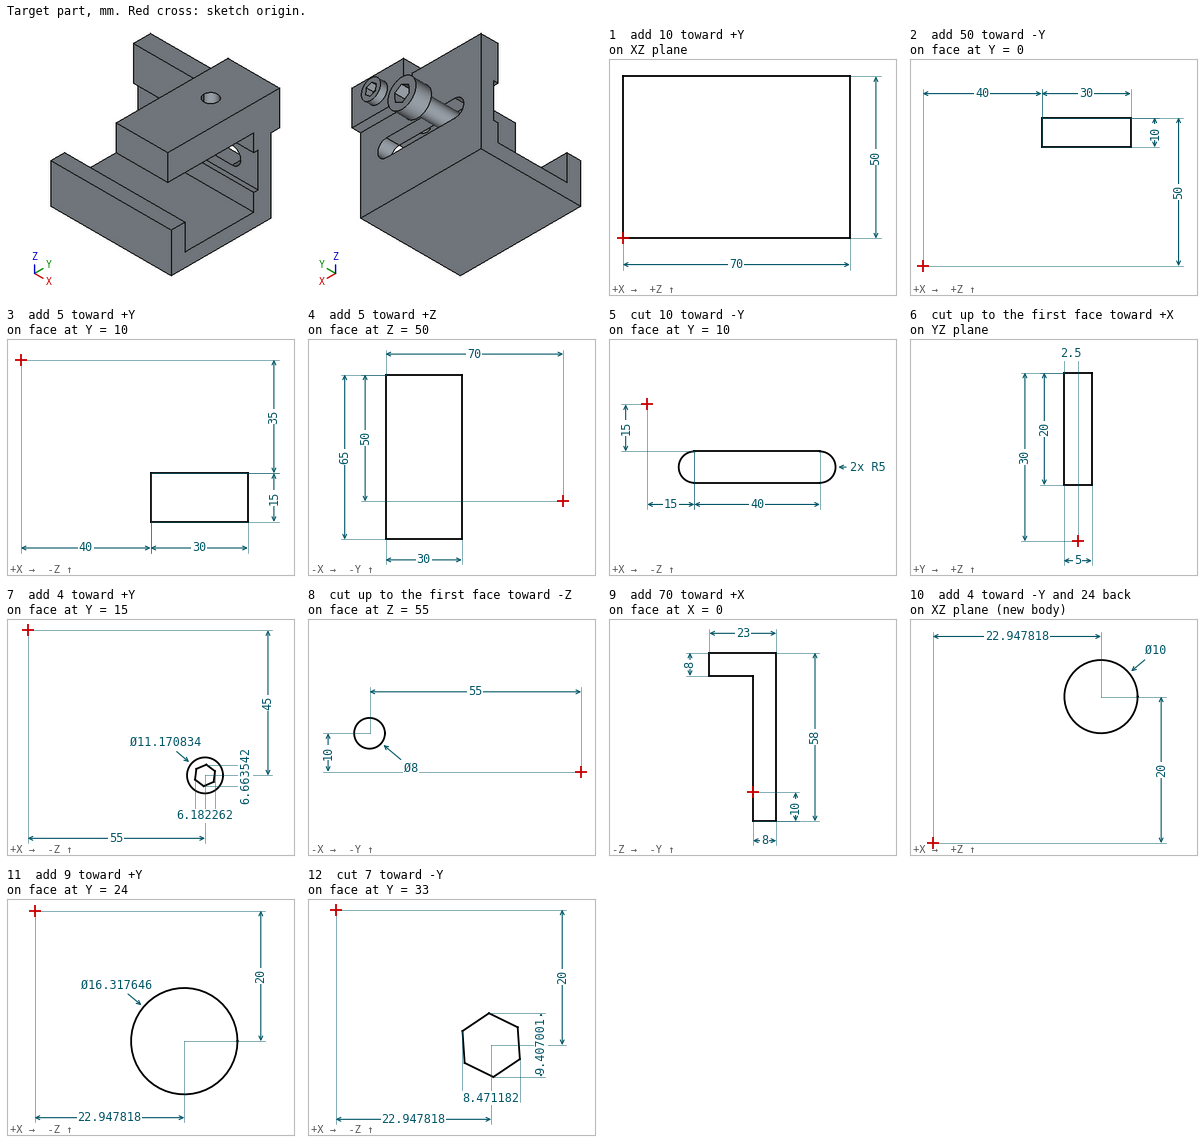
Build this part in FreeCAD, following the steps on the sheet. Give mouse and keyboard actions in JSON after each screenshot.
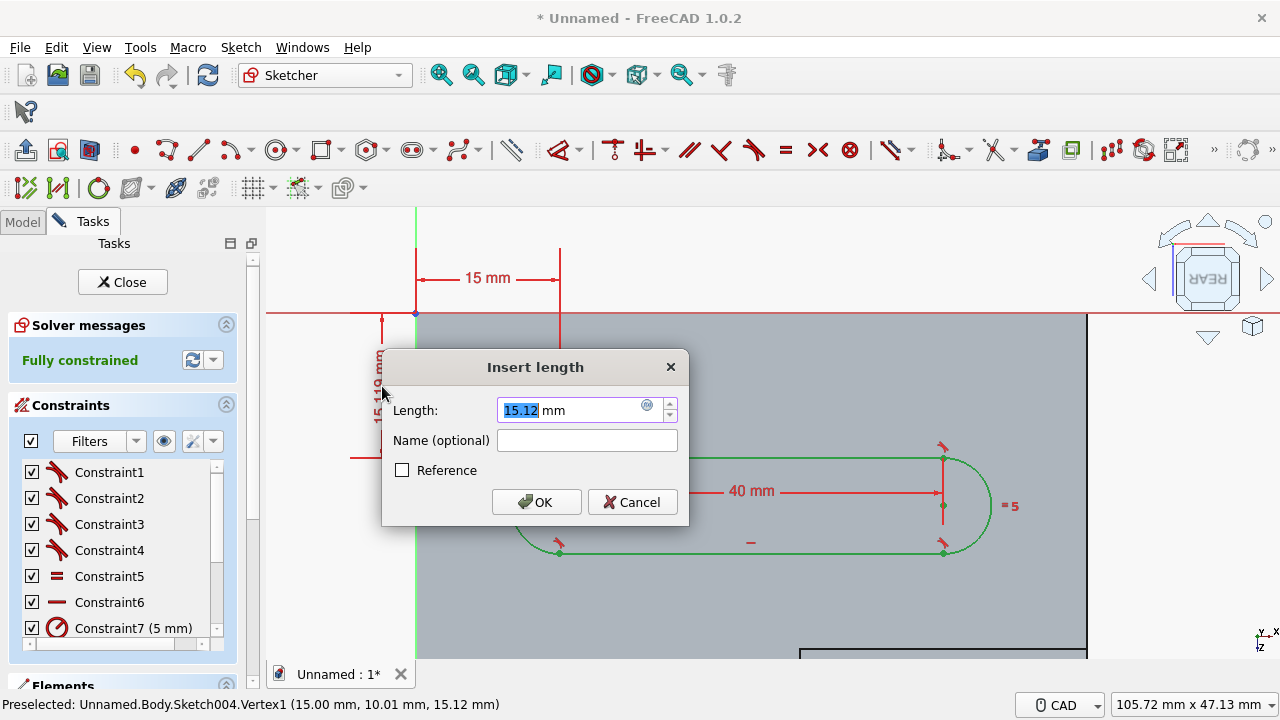
{"action": "type", "text": "15"}
{"action": "key", "text": "Return"}
{"action": "key", "text": "Escape"}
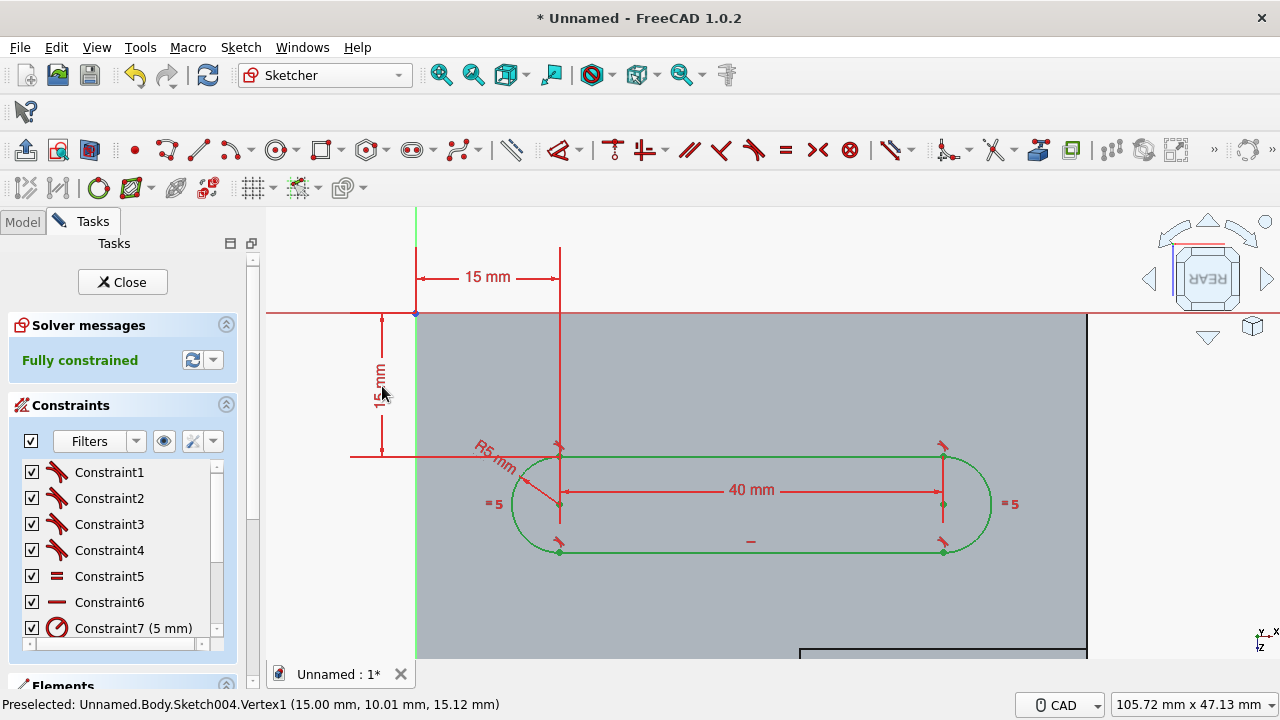
{"action": "left_click", "coordinate": [123, 282]}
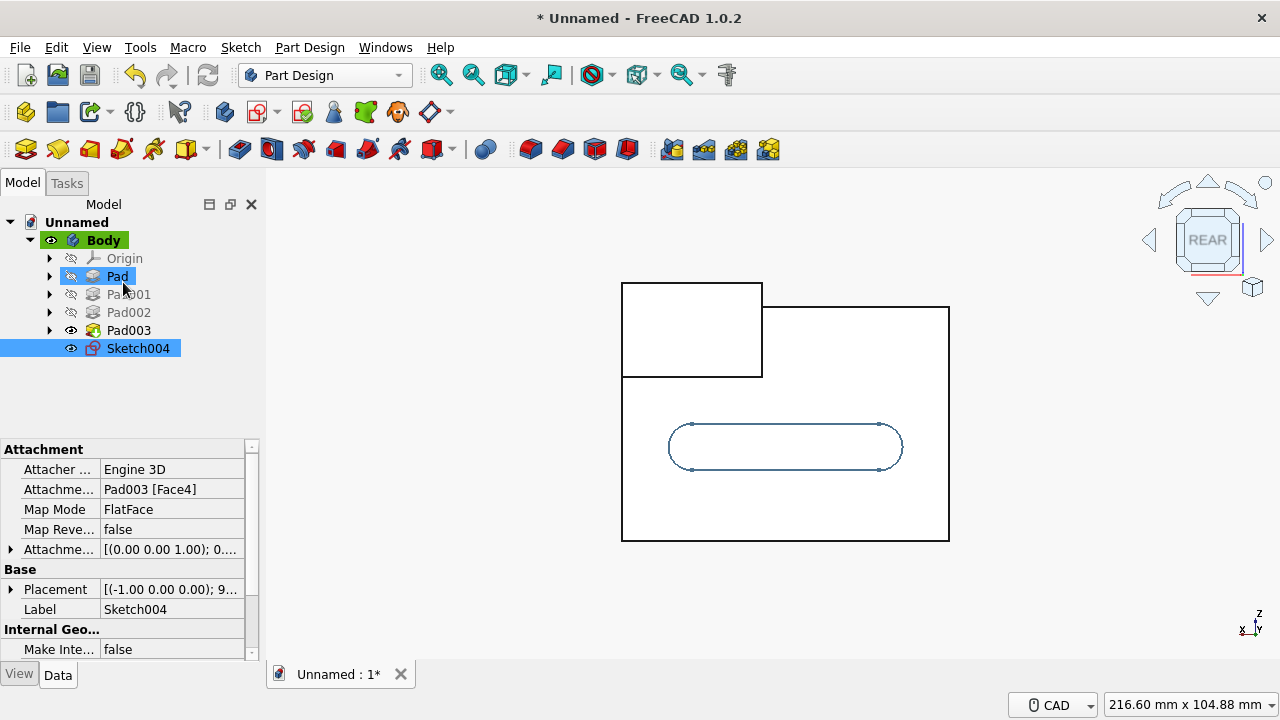
{"action": "left_click", "coordinate": [240, 150]}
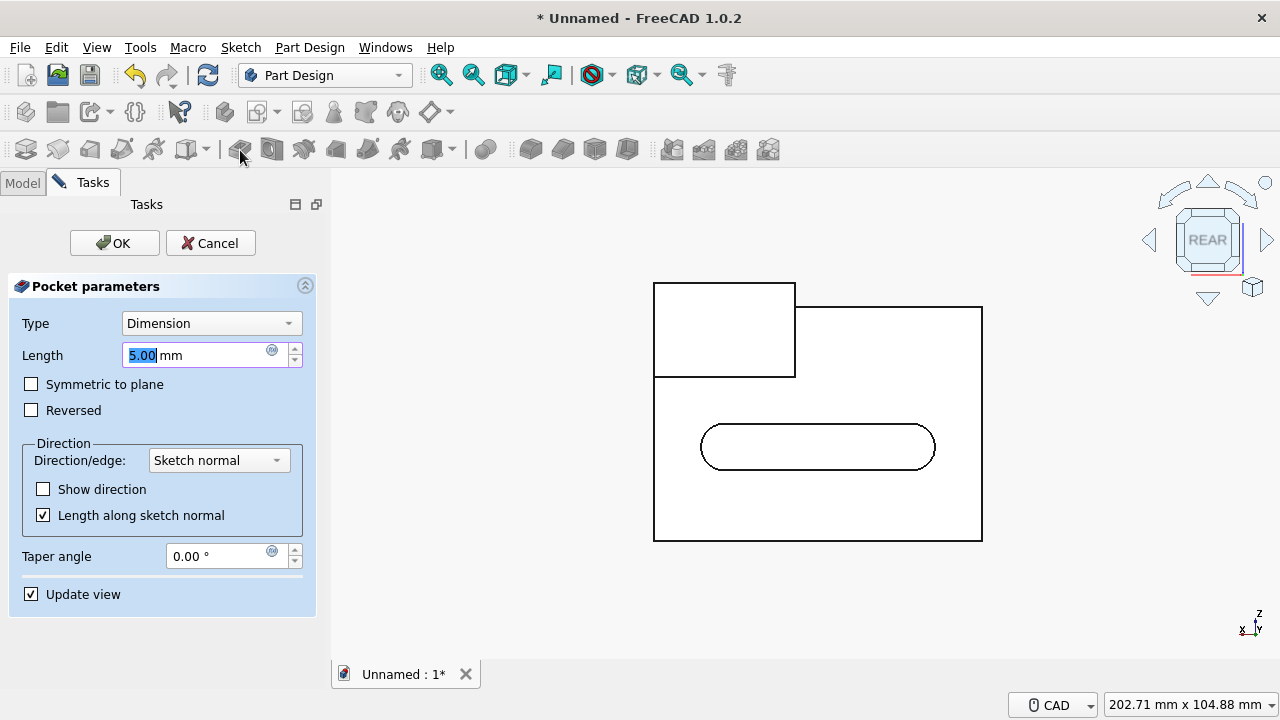
{"action": "type", "text": "10"}
{"action": "key", "text": "Tab"}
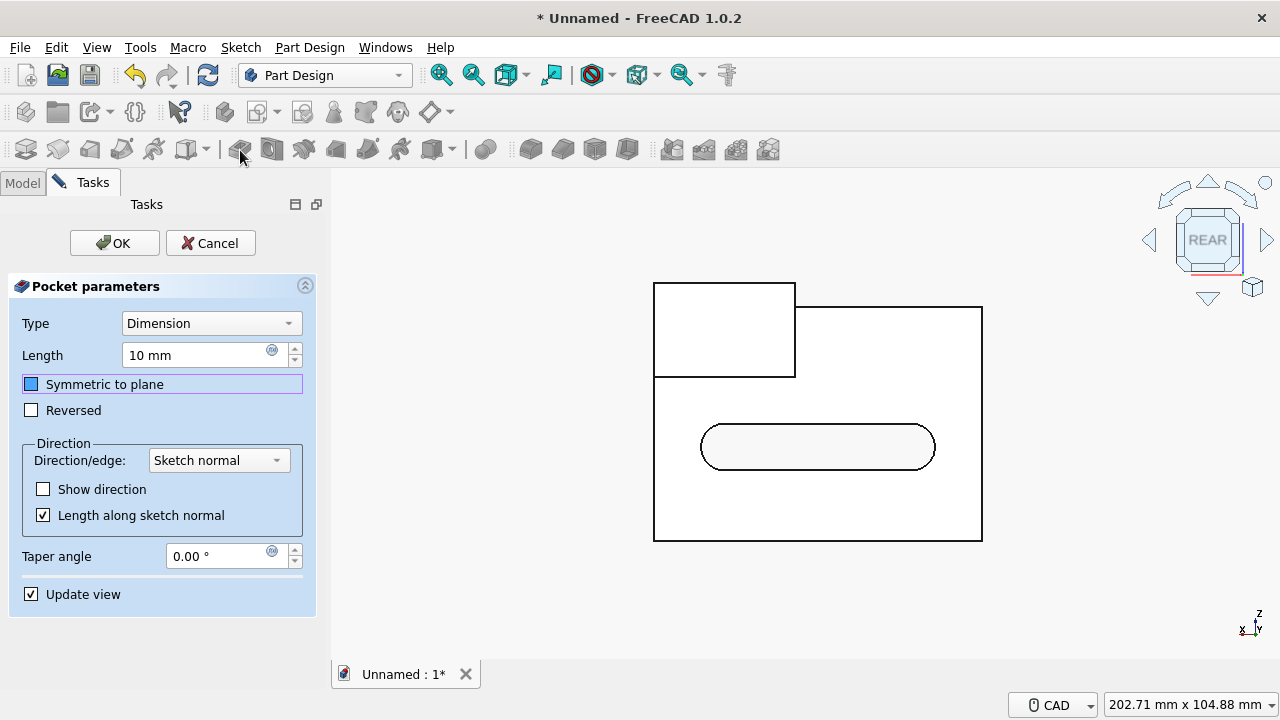
{"action": "left_click", "coordinate": [115, 243]}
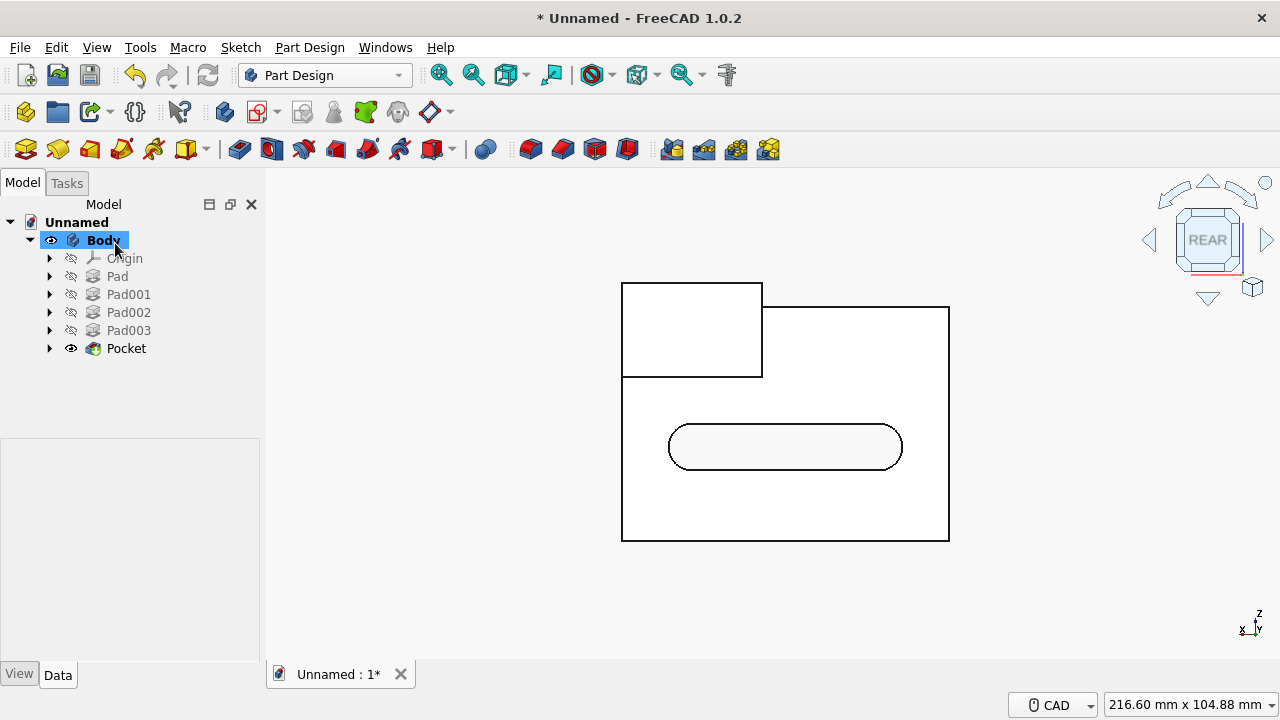
{"action": "left_click", "coordinate": [258, 112]}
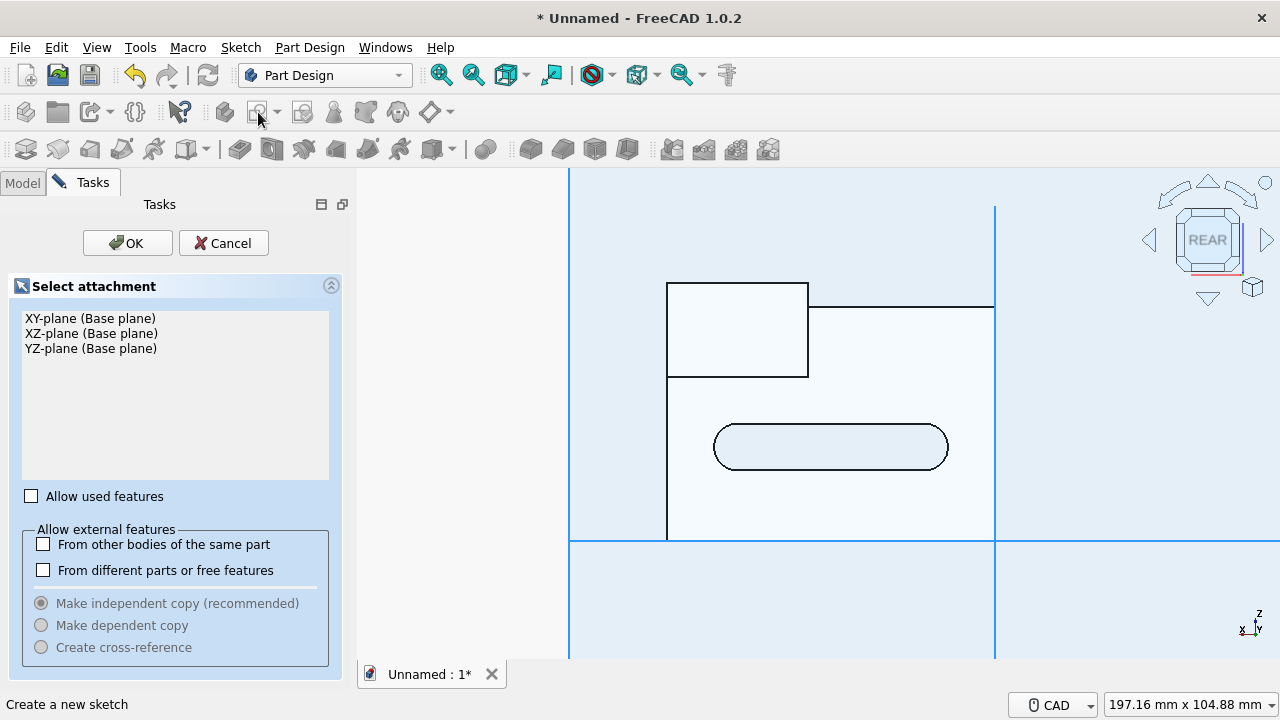
{"action": "left_click", "coordinate": [82, 348]}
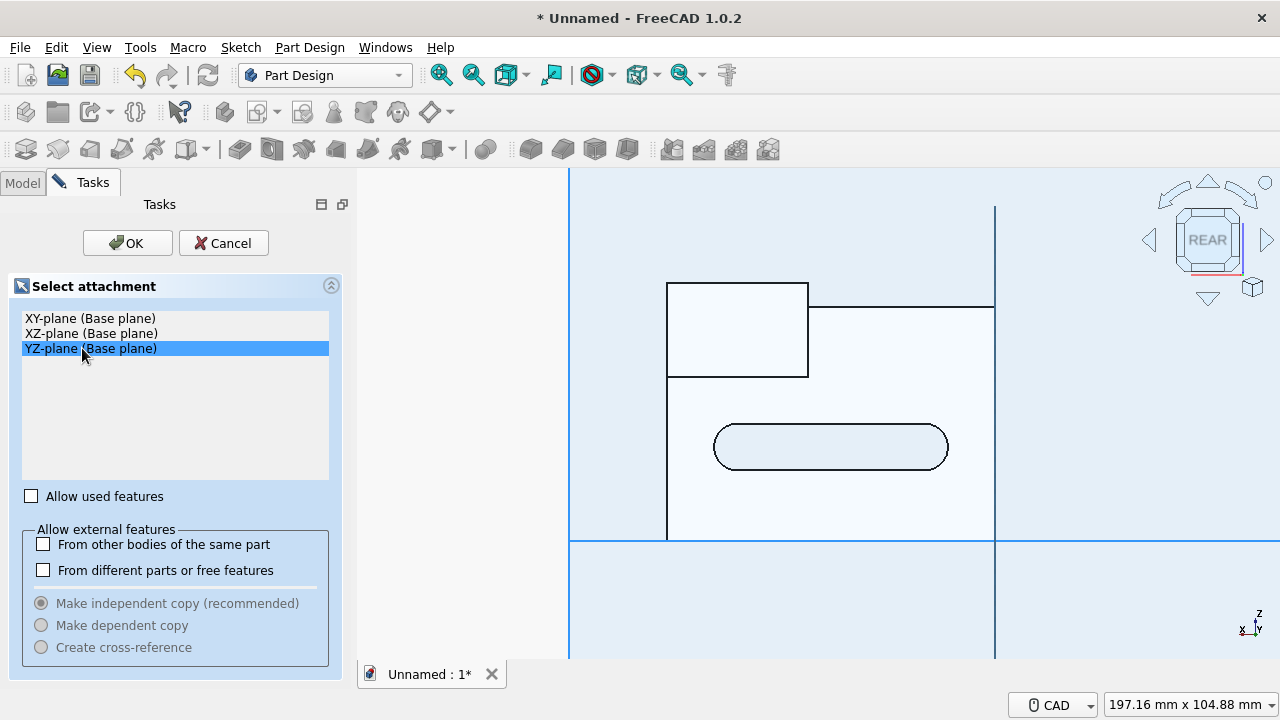
{"action": "left_click", "coordinate": [128, 243]}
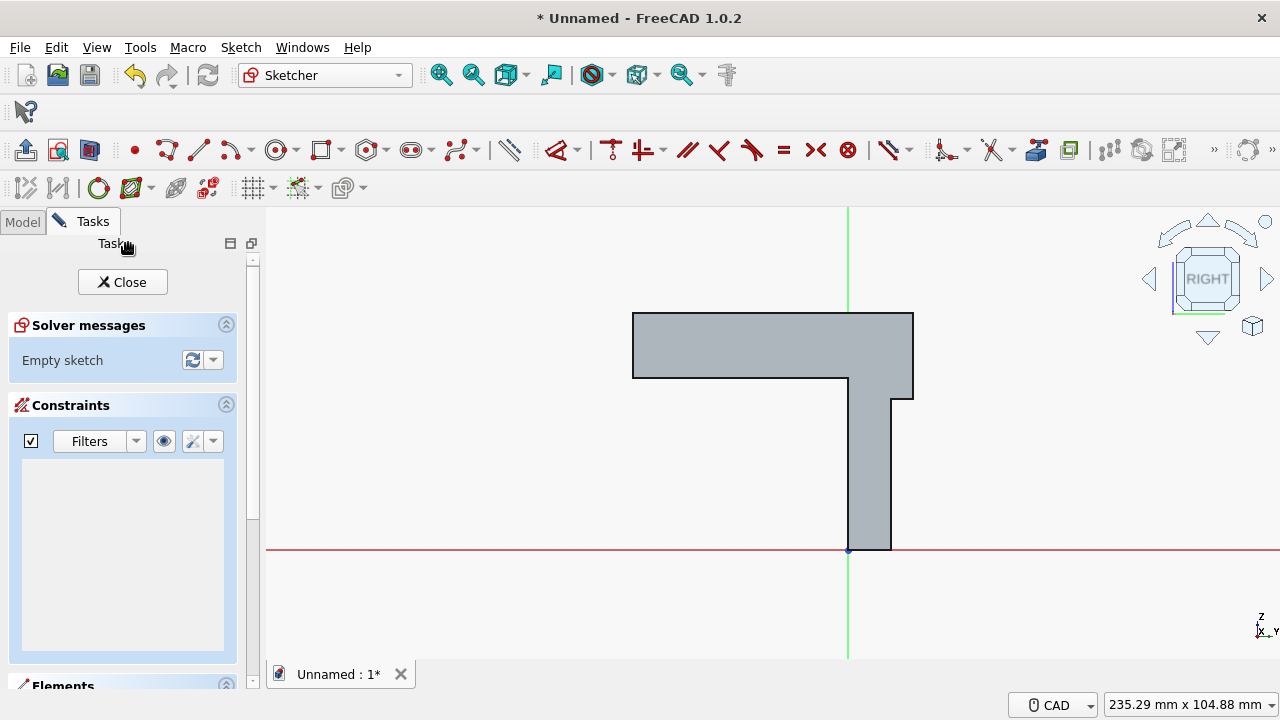
{"action": "left_click", "coordinate": [90, 150]}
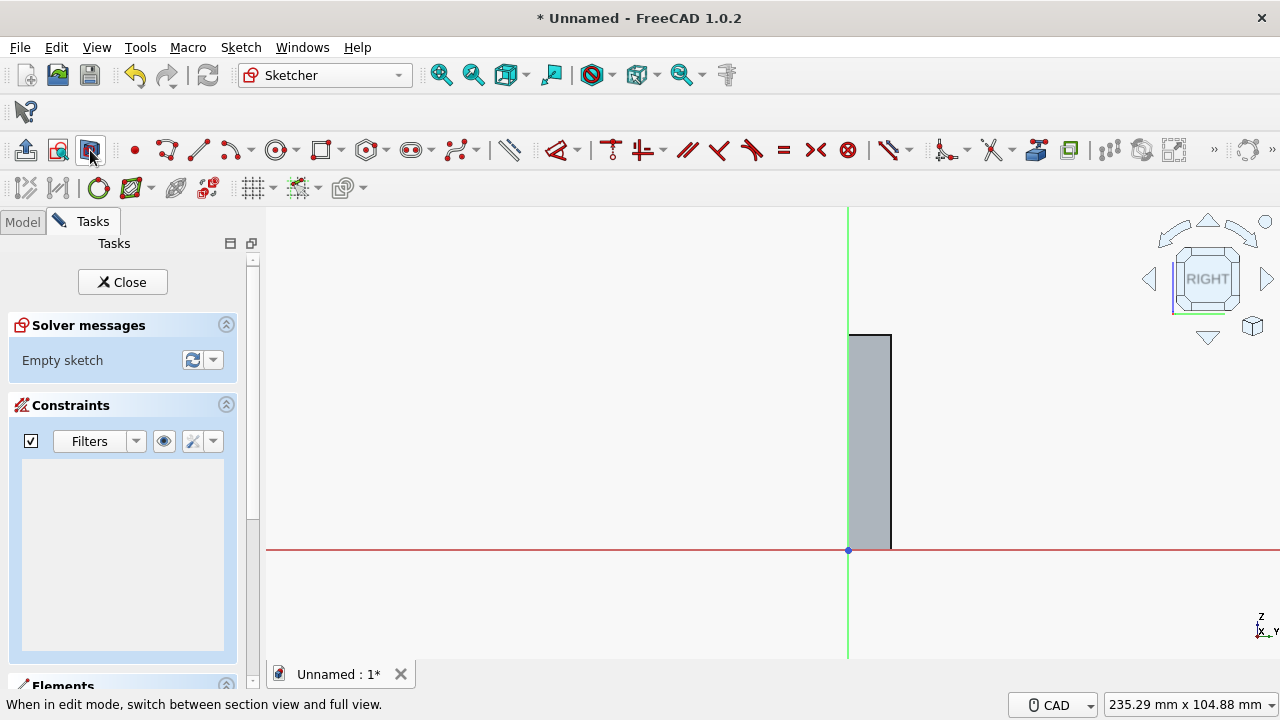
{"action": "scroll", "coordinate": [965, 528], "scroll_direction": "up", "scroll_amount": 4}